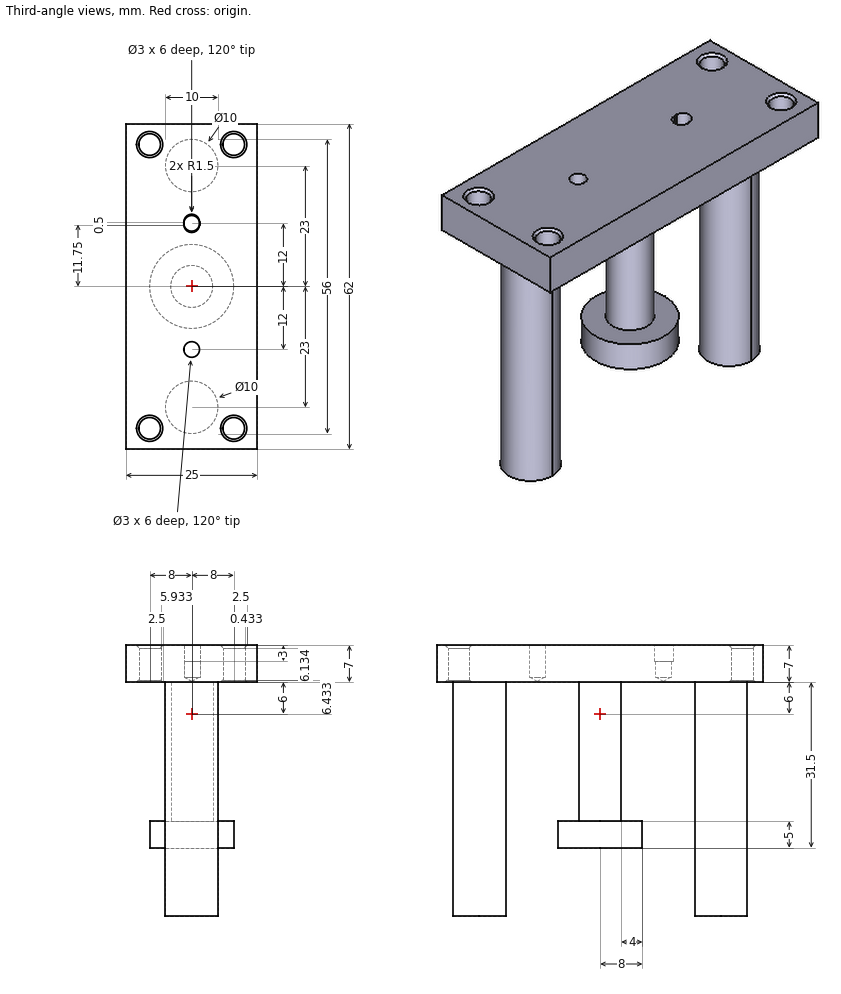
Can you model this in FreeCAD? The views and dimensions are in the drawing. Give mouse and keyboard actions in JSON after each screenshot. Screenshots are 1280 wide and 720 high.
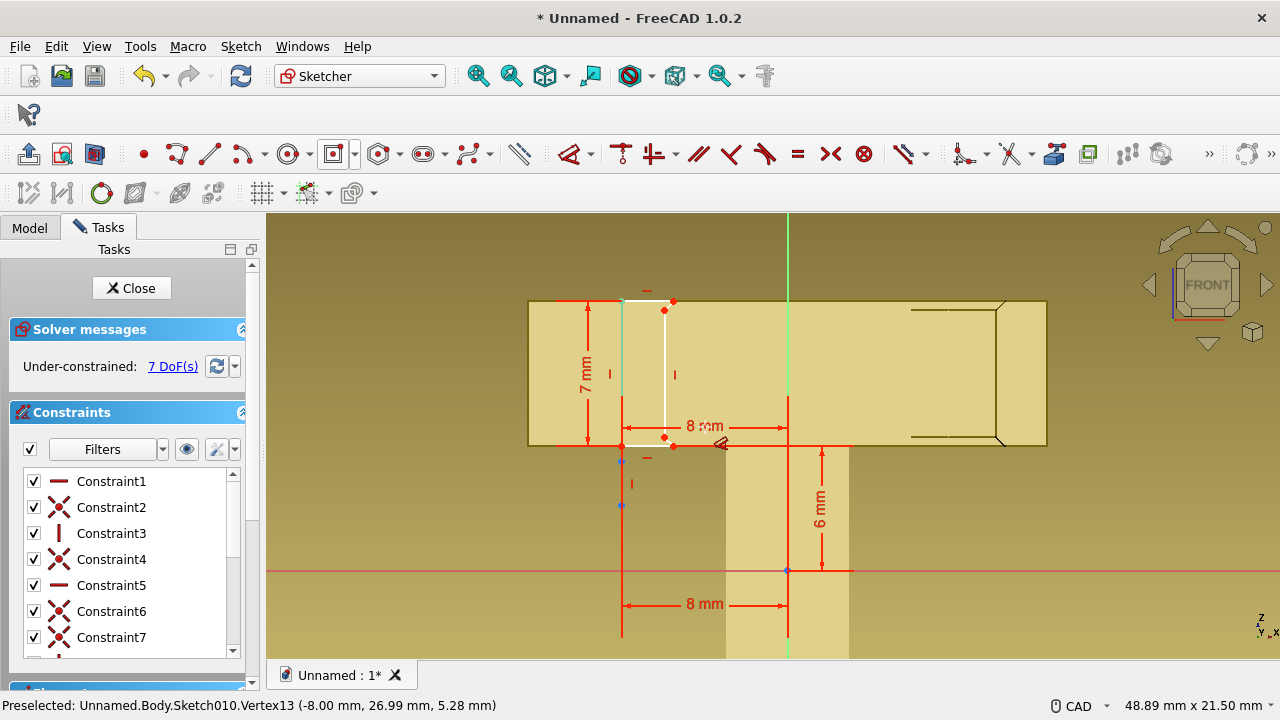
{"action": "scroll", "coordinate": [658, 446], "scroll_direction": "up", "scroll_amount": 2}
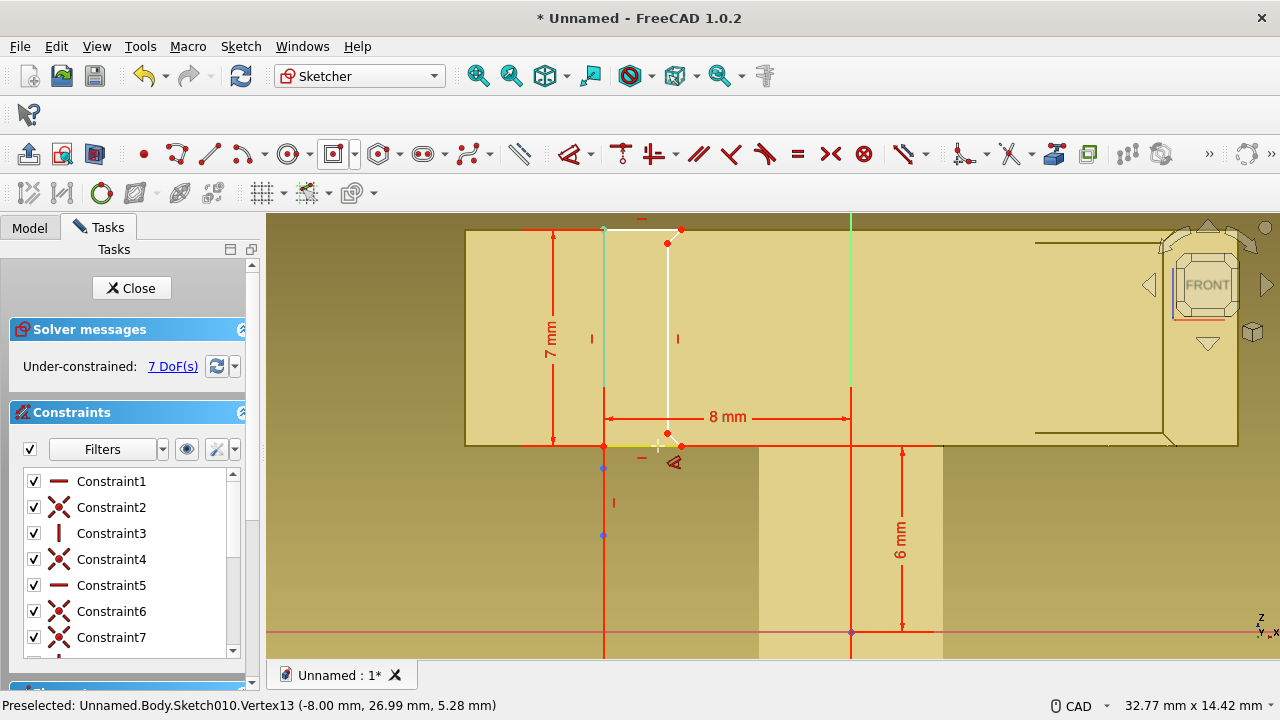
{"action": "left_click", "coordinate": [658, 446]}
{"action": "left_click", "coordinate": [643, 480]}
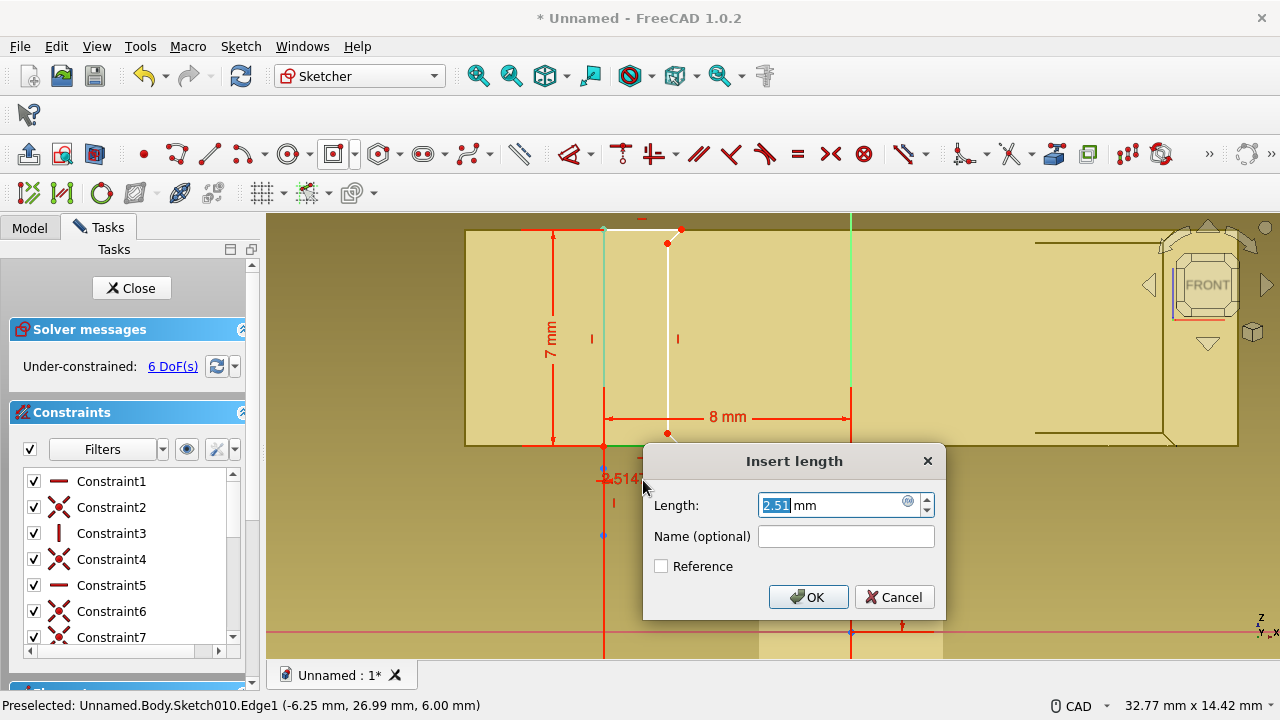
{"action": "type", "text": "2.5"}
{"action": "key", "text": "Return"}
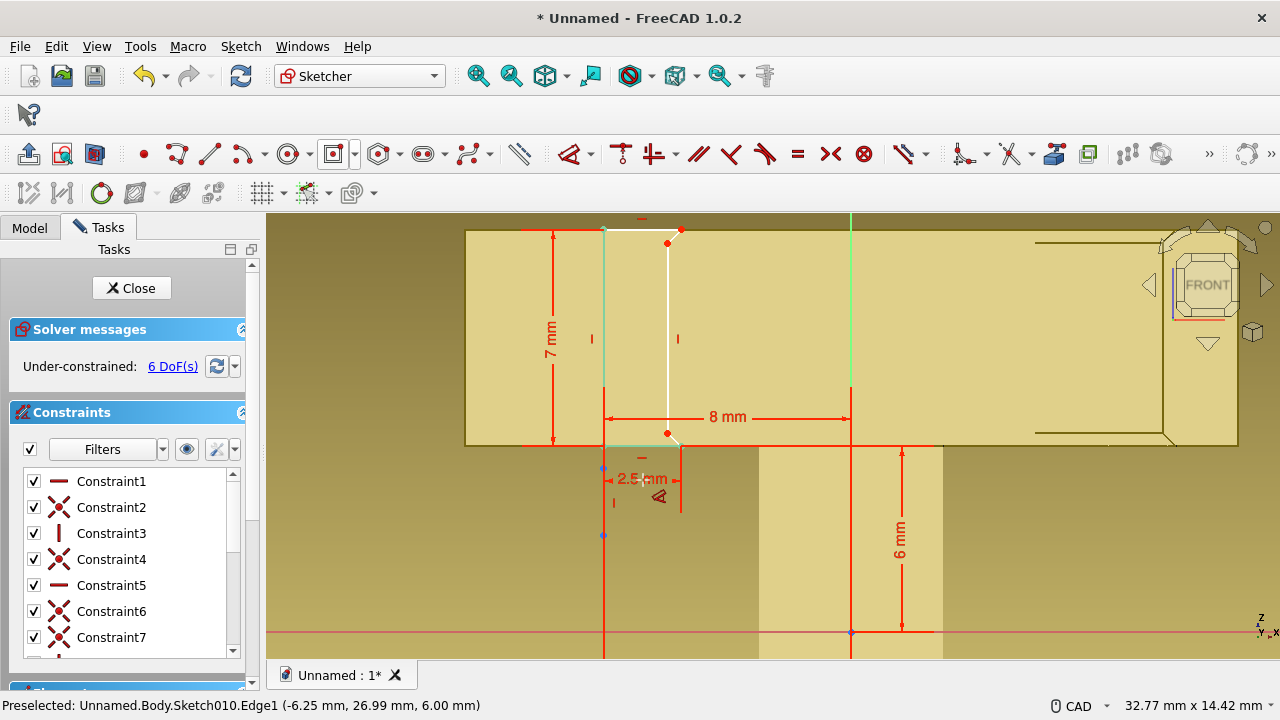
{"action": "scroll", "coordinate": [658, 446], "scroll_direction": "down", "scroll_amount": 2}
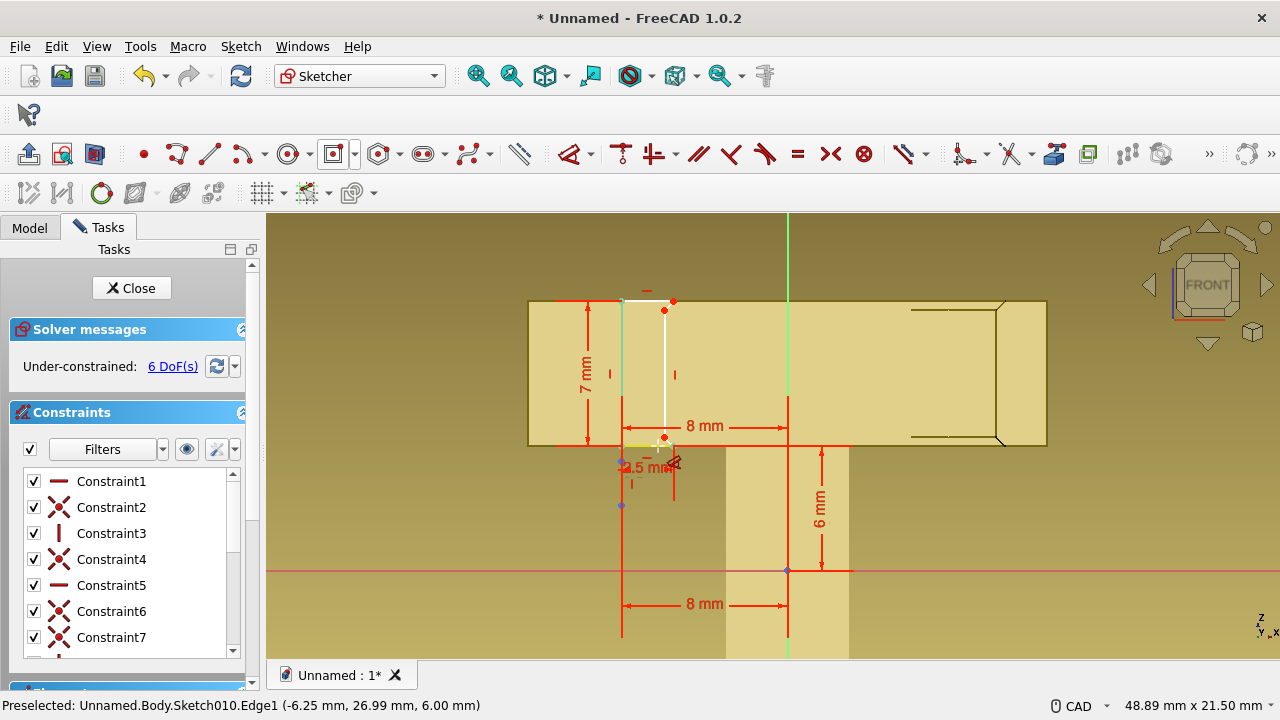
{"action": "left_click", "coordinate": [637, 301]}
{"action": "left_click", "coordinate": [648, 267]}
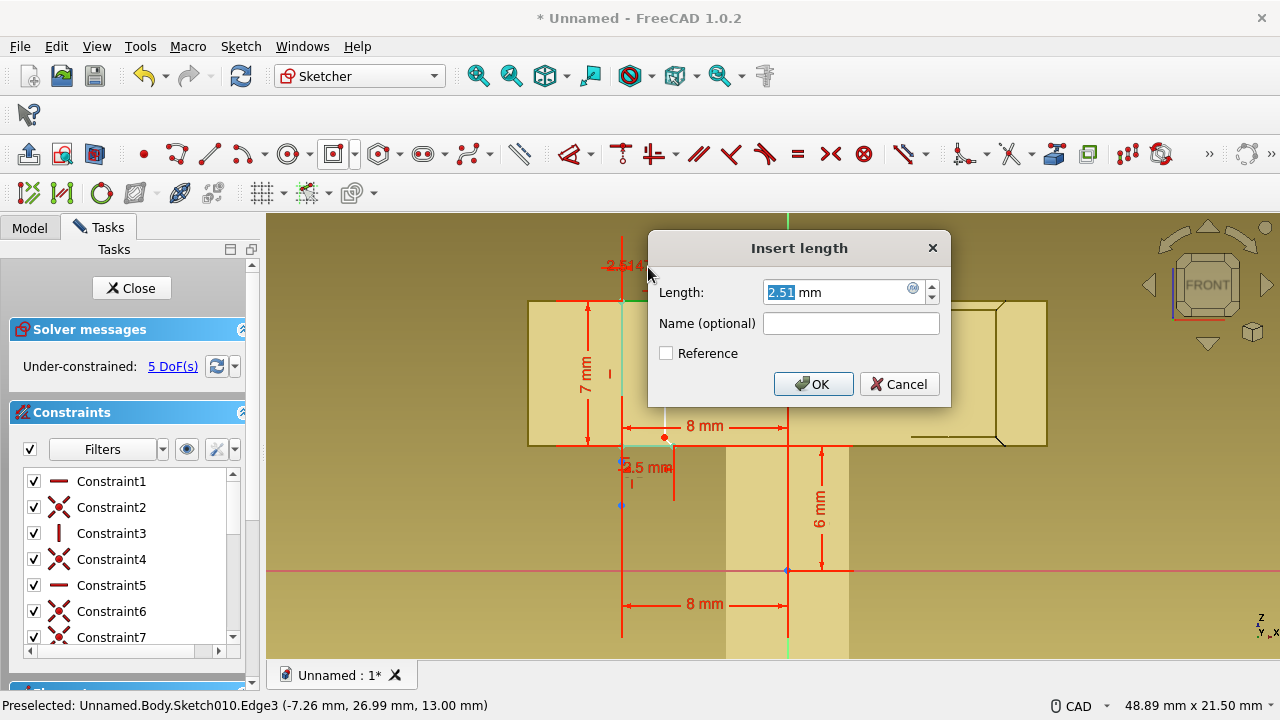
{"action": "type", "text": "2.5"}
{"action": "key", "text": "Return"}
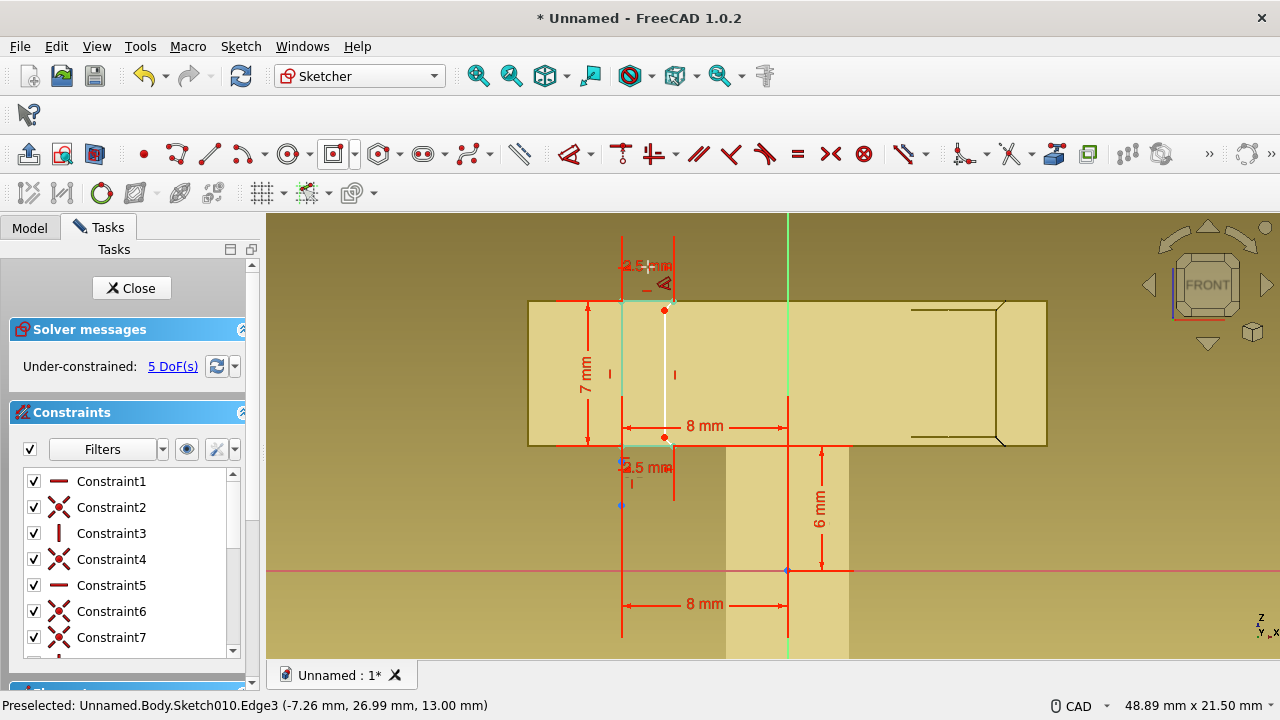
{"action": "left_click", "coordinate": [665, 349]}
{"action": "left_click", "coordinate": [699, 374]}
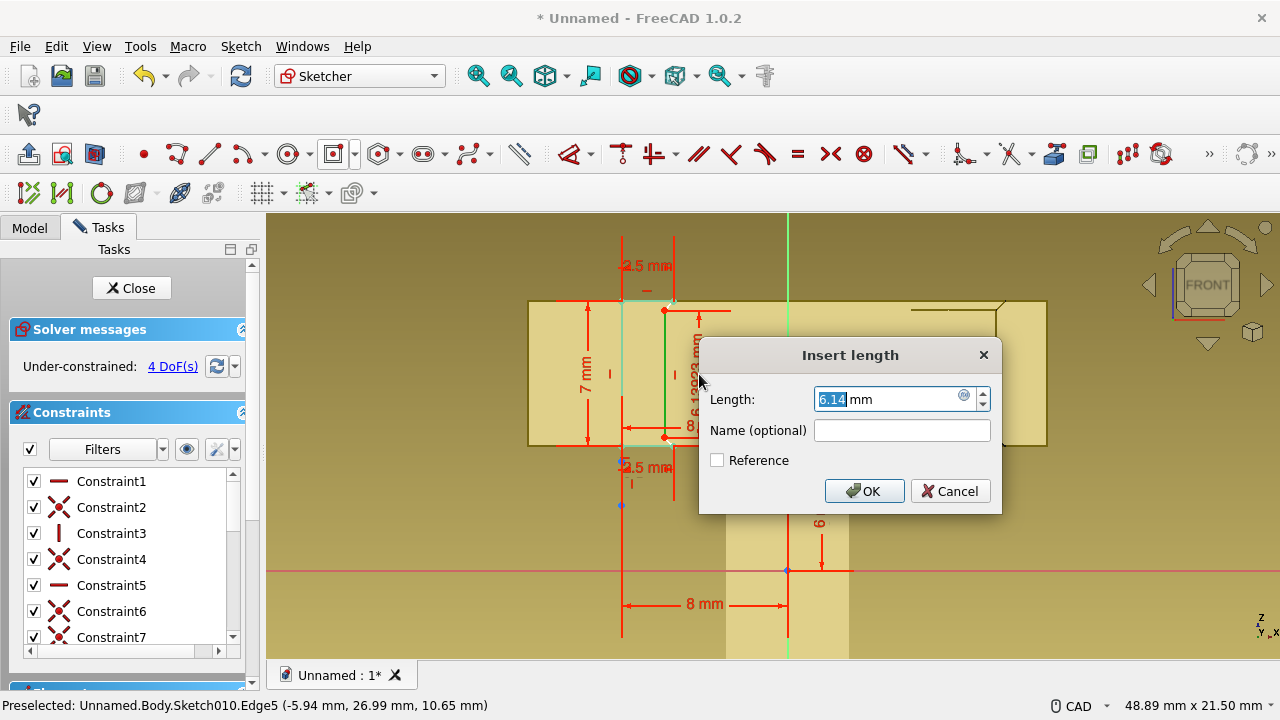
{"action": "type", "text": "6.134"}
{"action": "key", "text": "Return"}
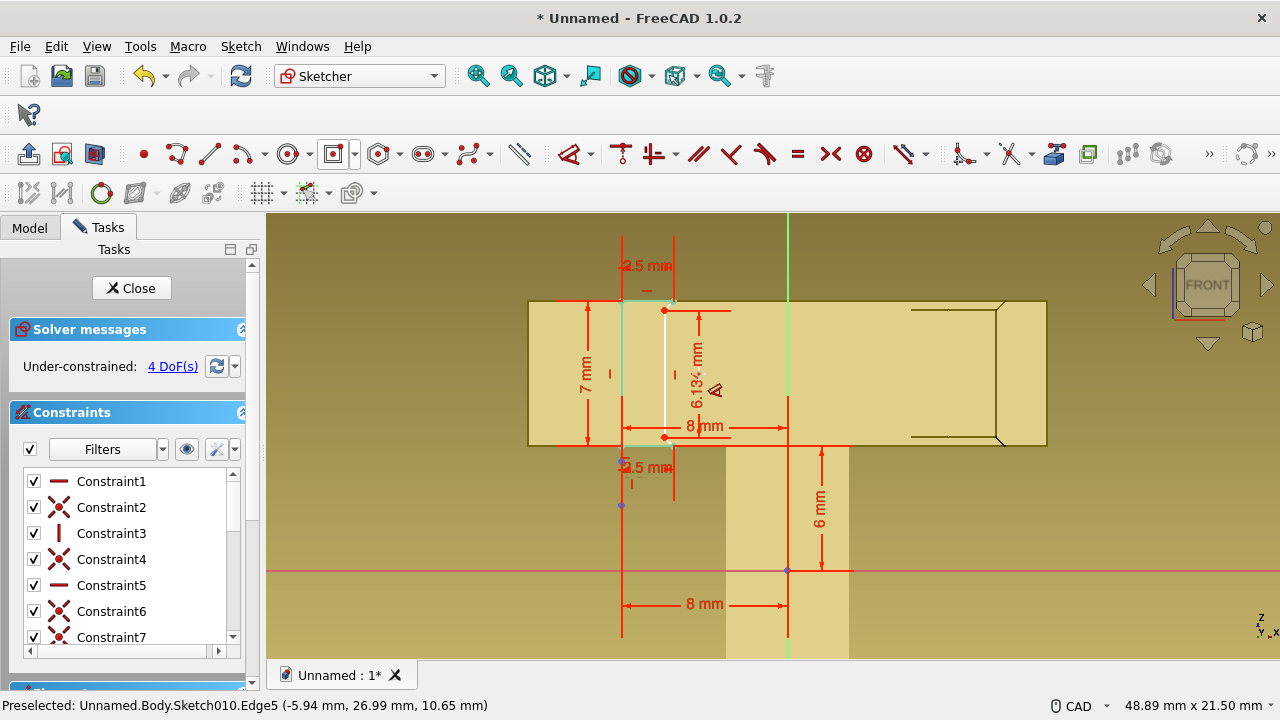
{"action": "left_click", "coordinate": [665, 311]}
{"action": "left_click", "coordinate": [726, 277]}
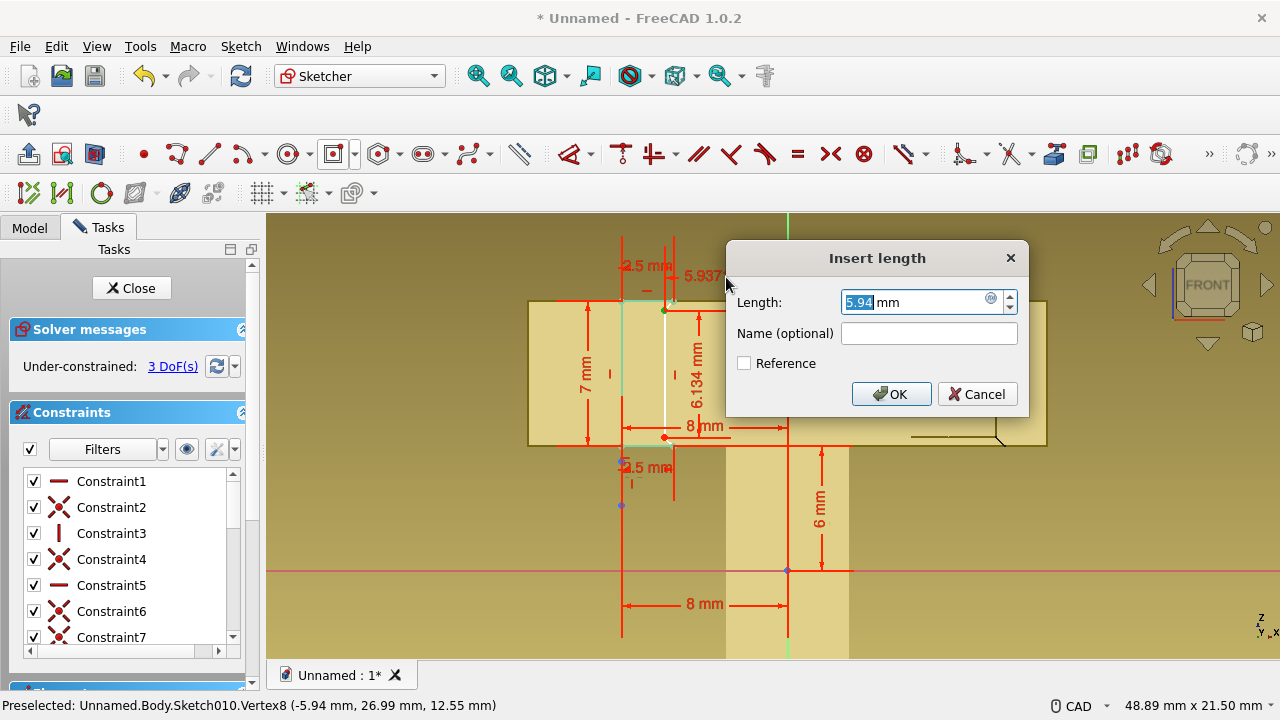
{"action": "type", "text": "5.933"}
{"action": "key", "text": "Return"}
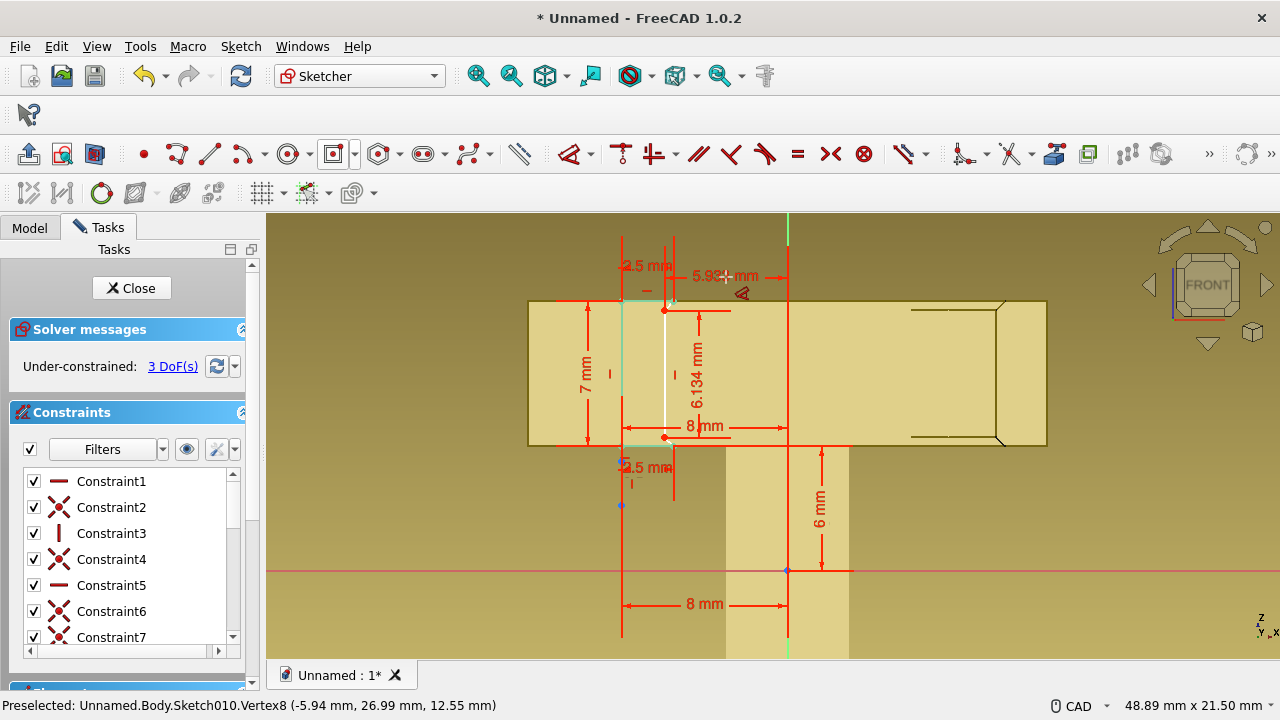
{"action": "left_click", "coordinate": [665, 438]}
{"action": "left_click", "coordinate": [822, 474]}